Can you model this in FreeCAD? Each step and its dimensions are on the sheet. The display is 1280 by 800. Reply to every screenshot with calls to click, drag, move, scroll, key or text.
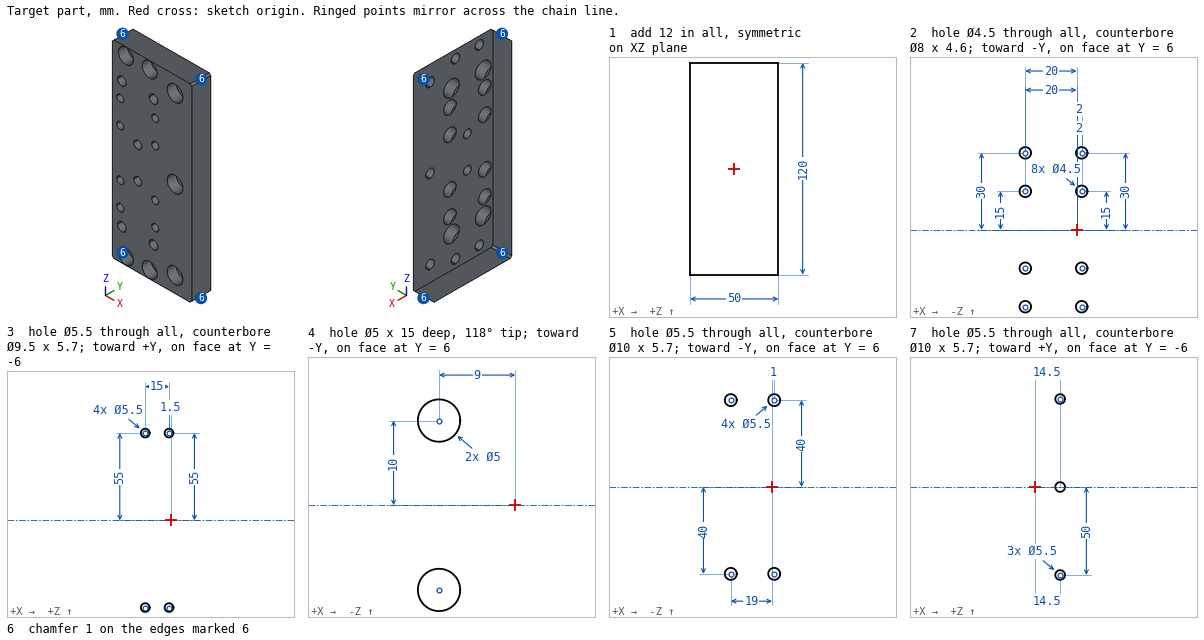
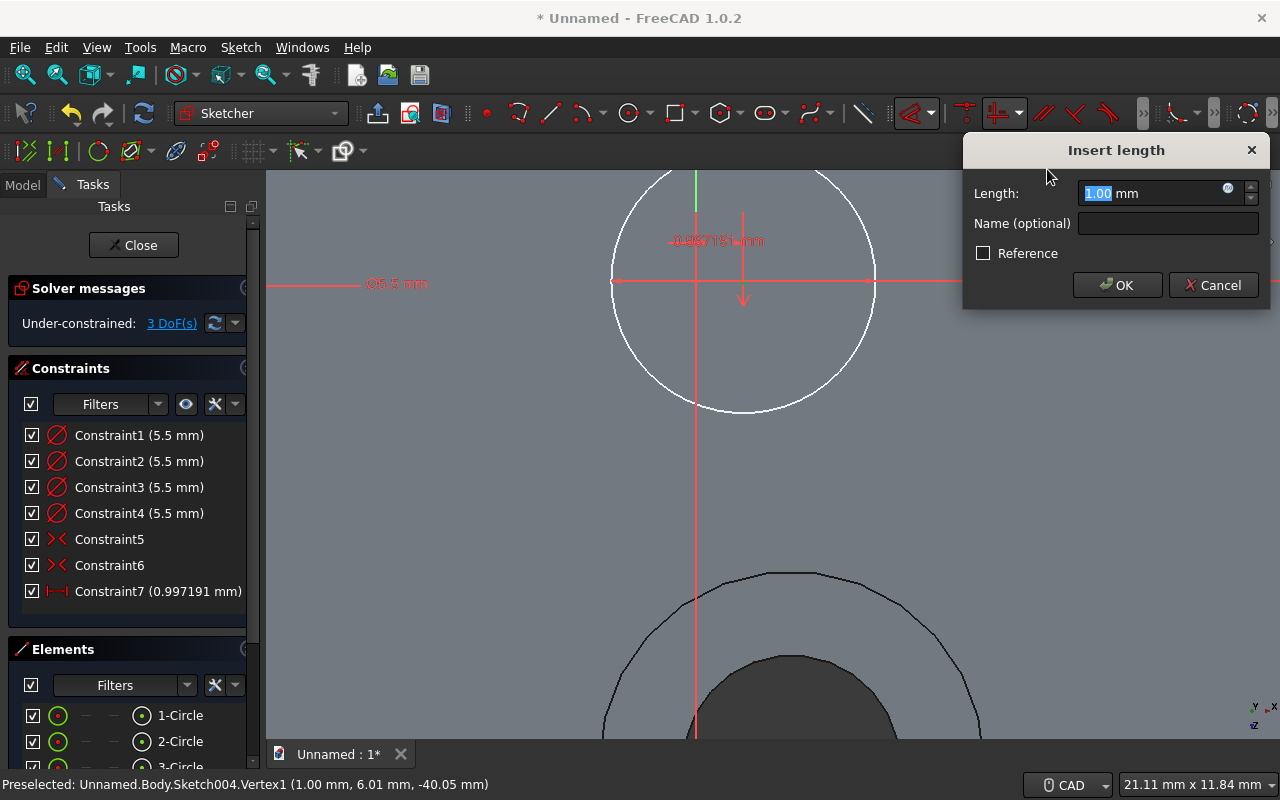
text(1)
key(Return)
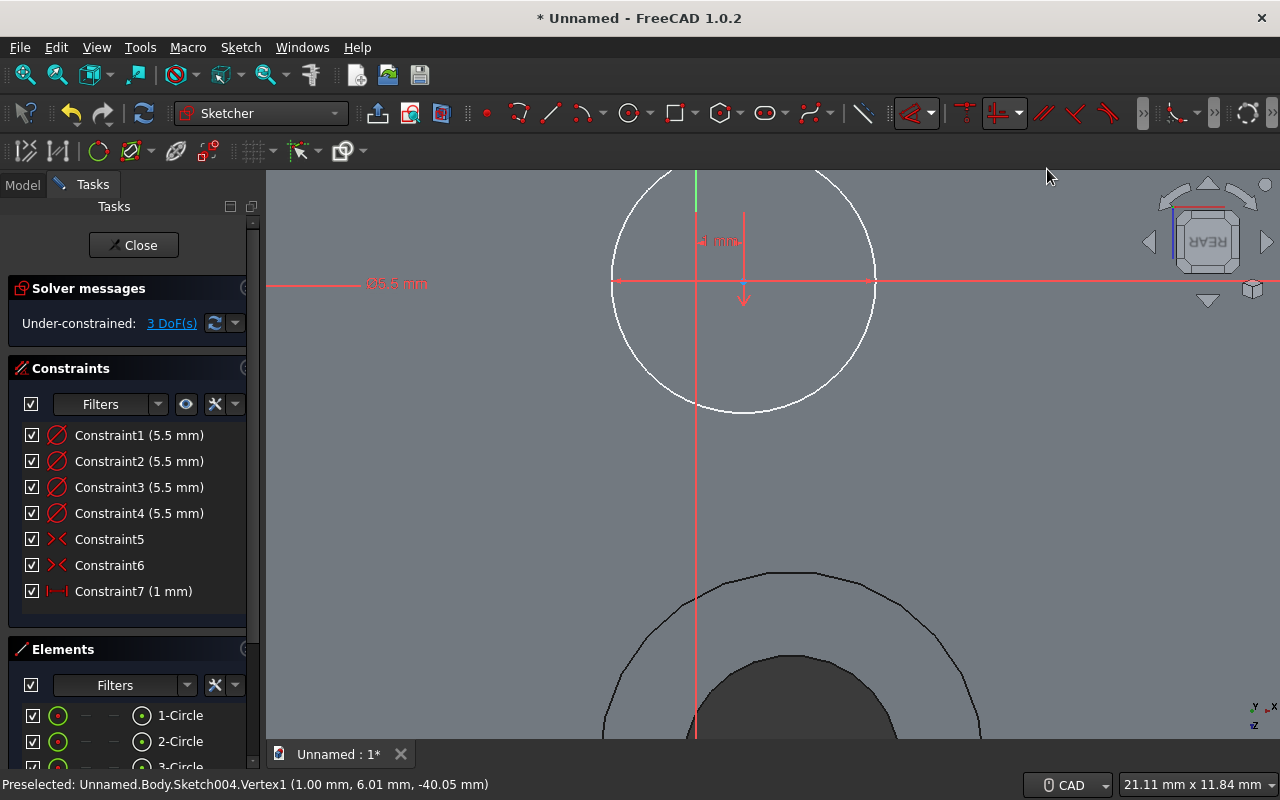
scroll(749, 280, down, 12)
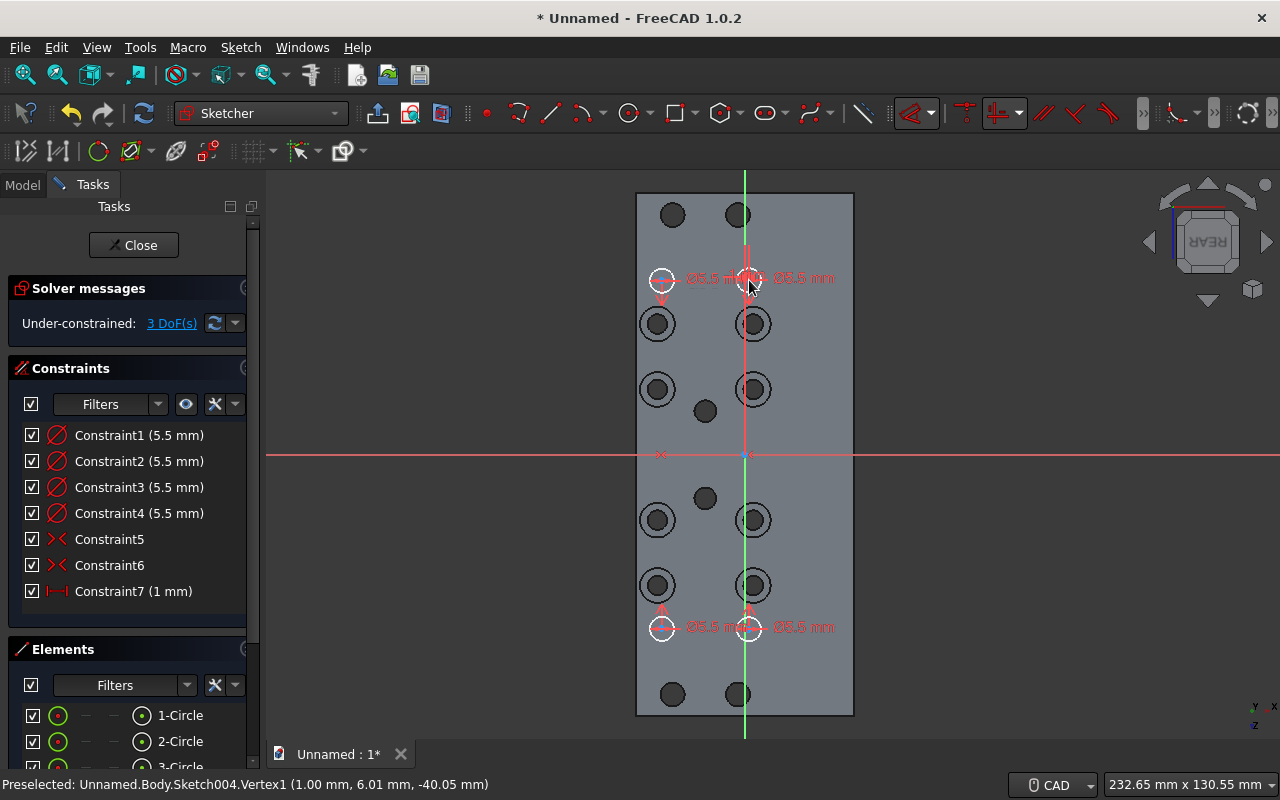
click(749, 280)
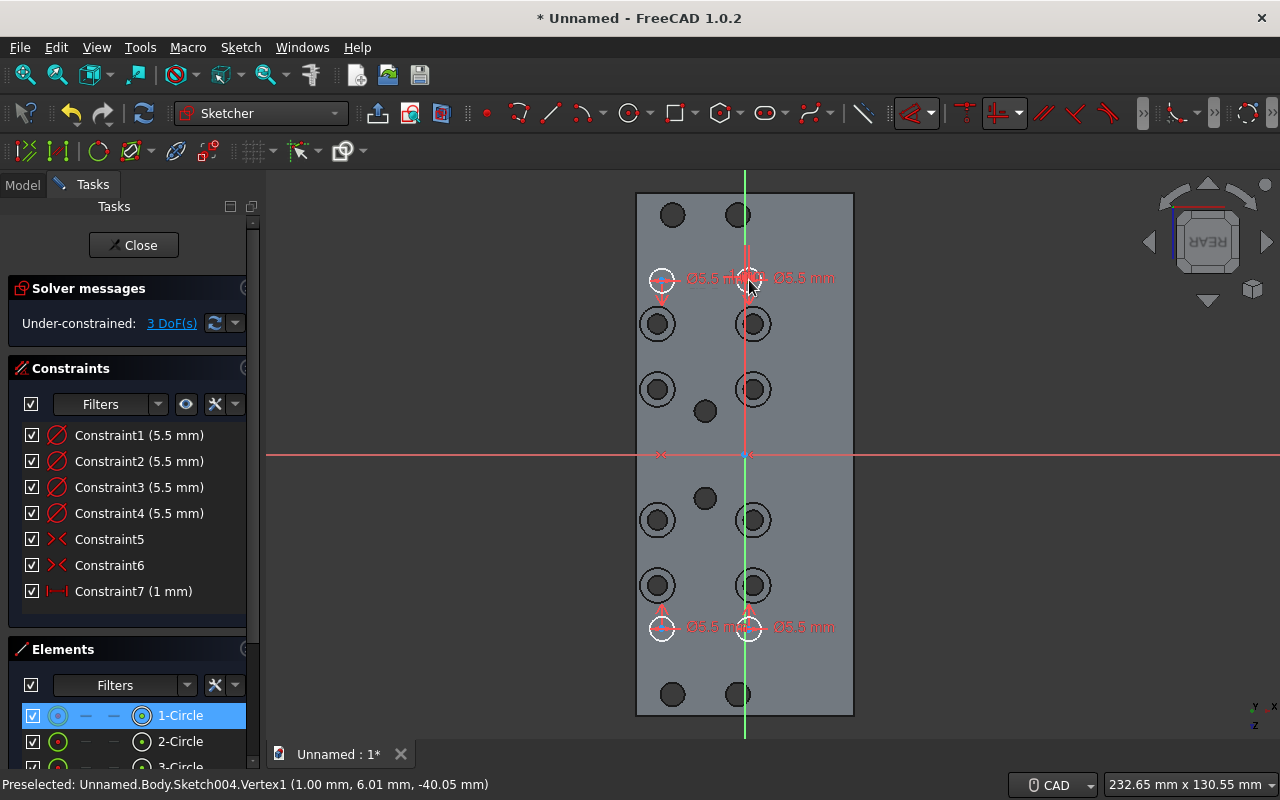
click(934, 114)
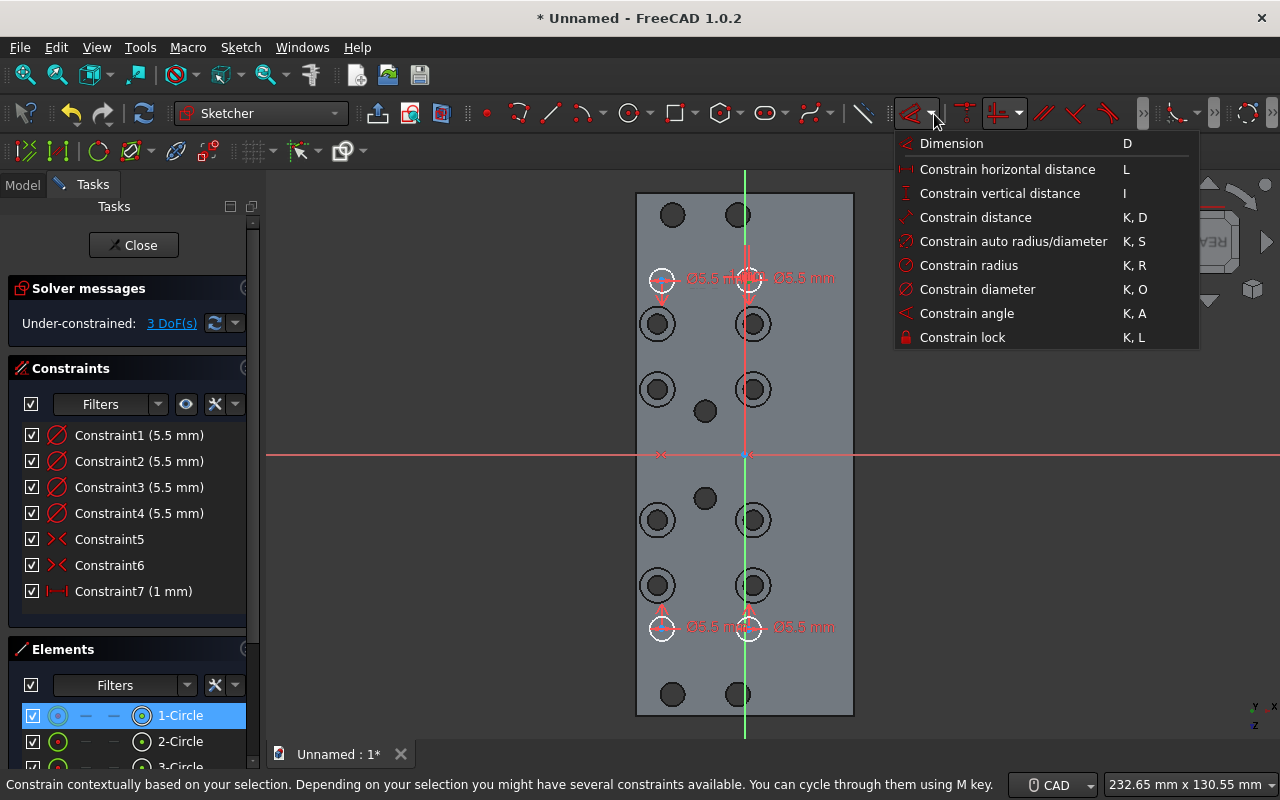
click(1047, 193)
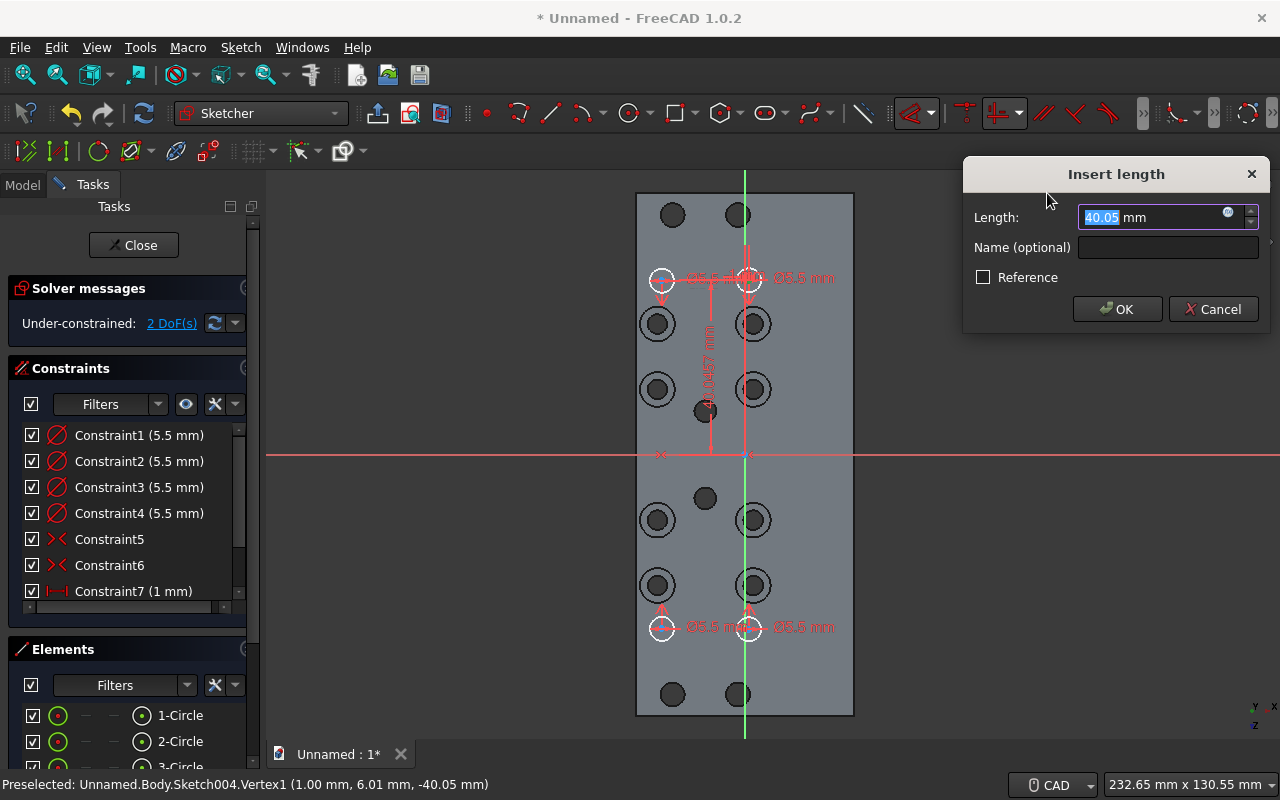
text(40)
key(Return)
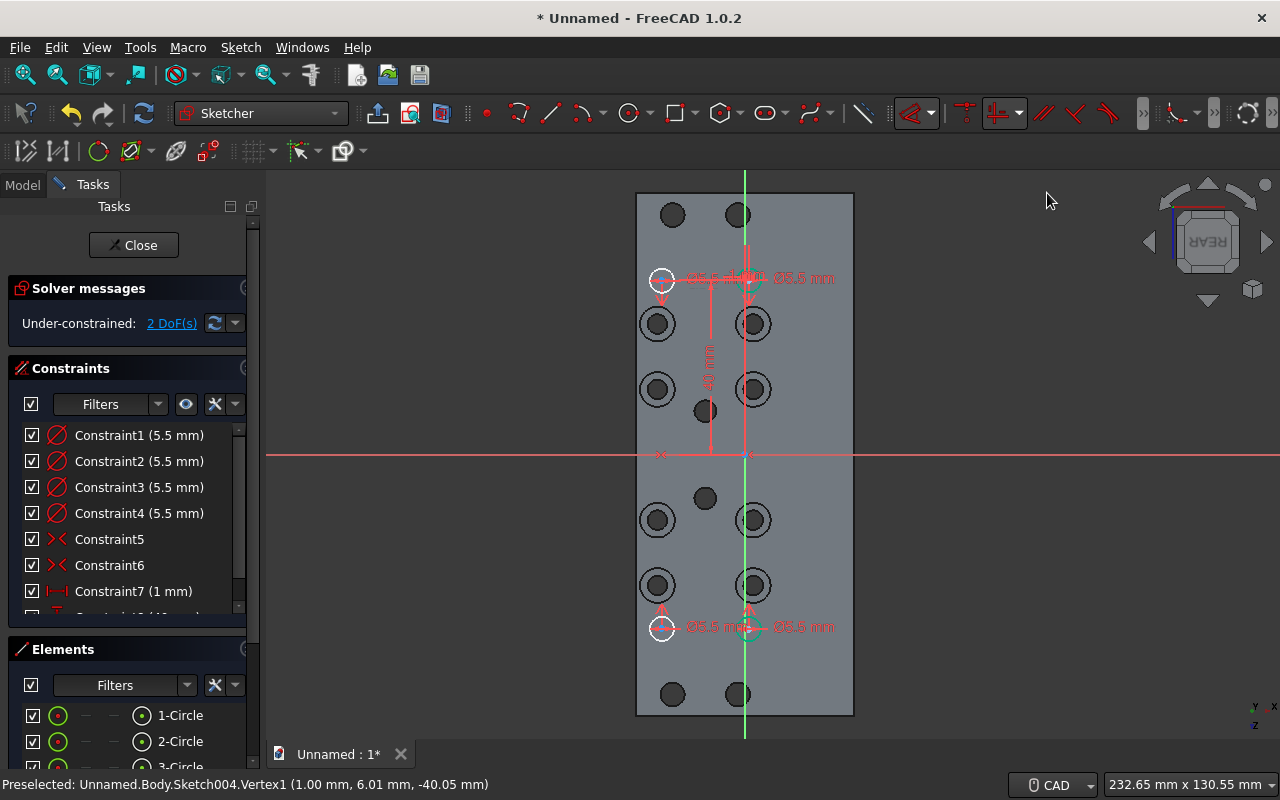
click(662, 629)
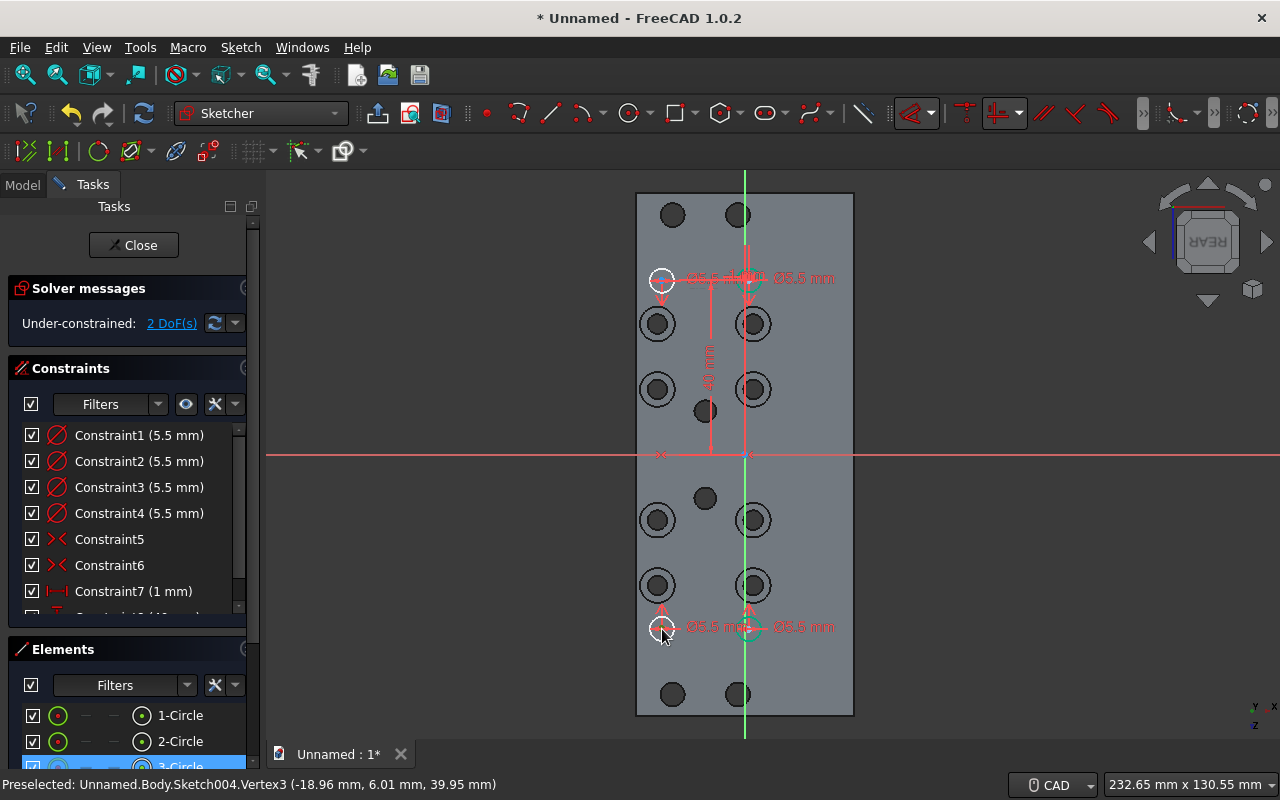
key(l)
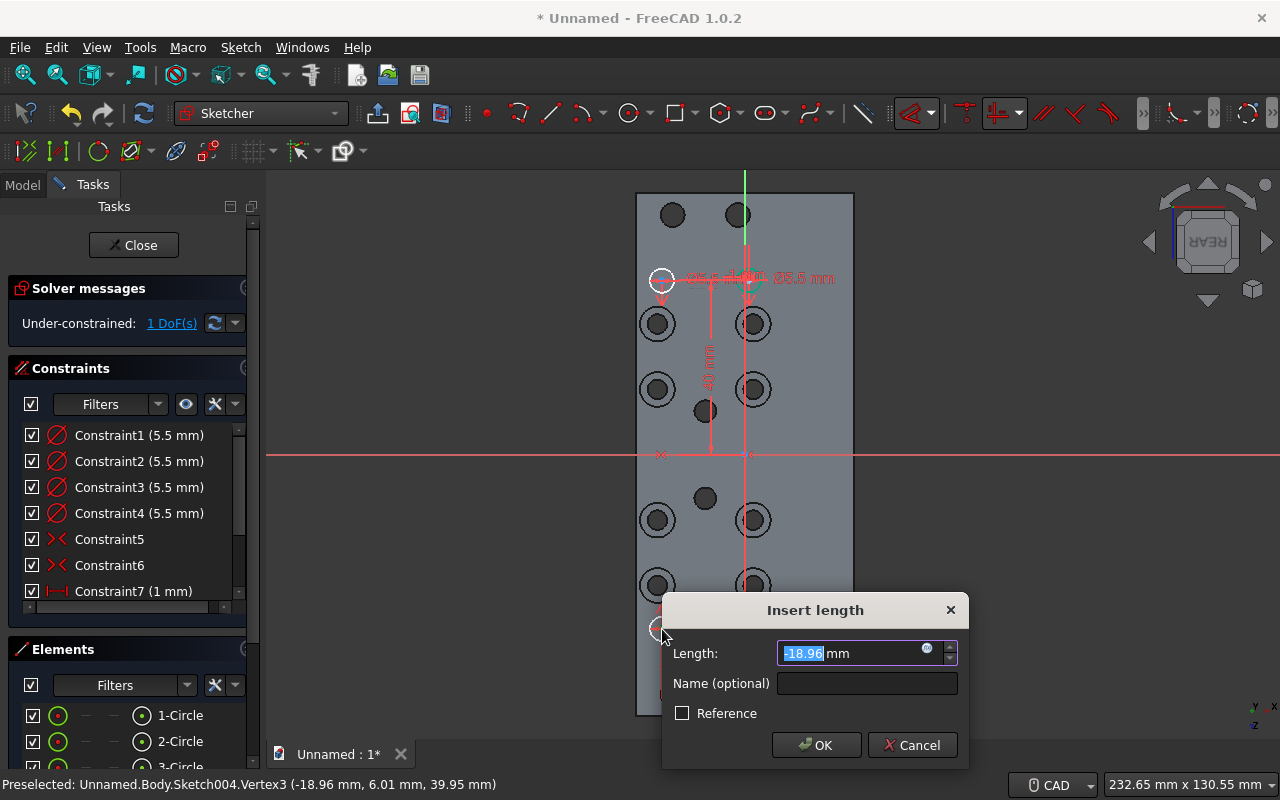
text(-19)
key(Return)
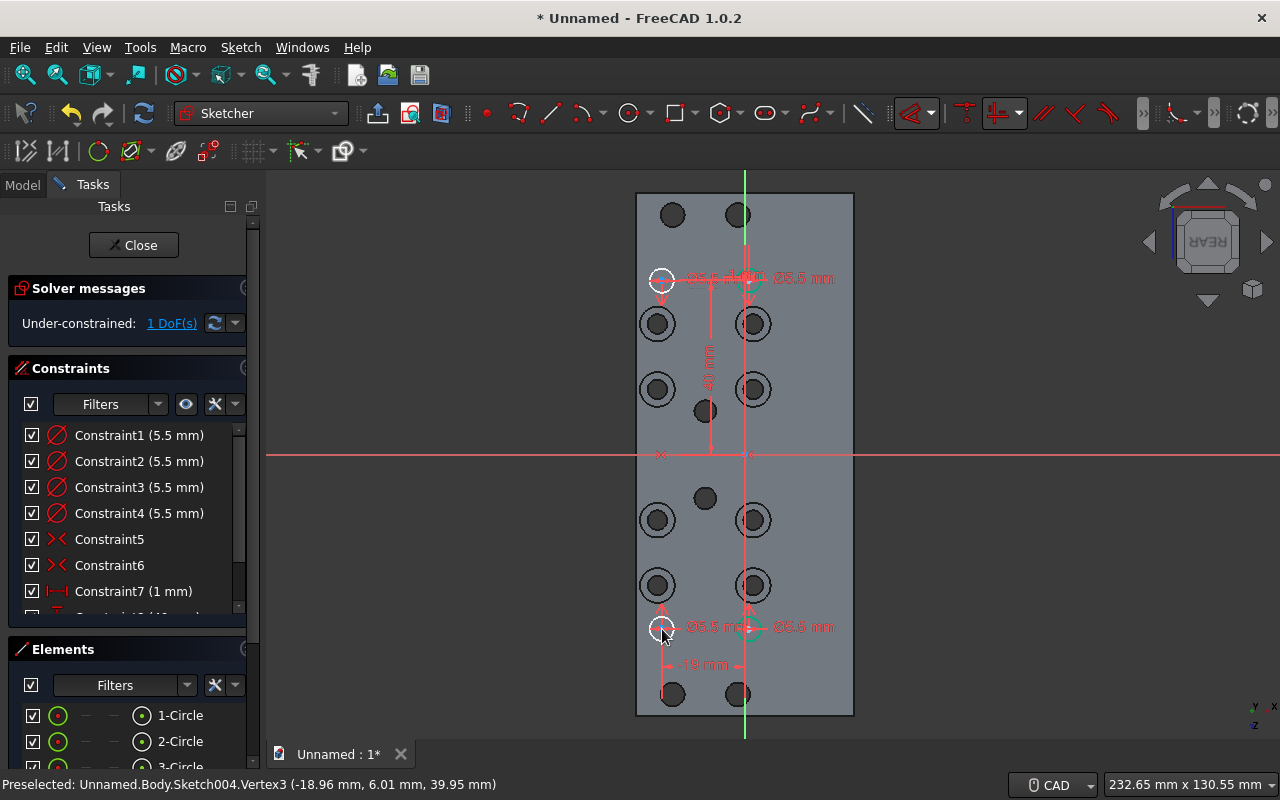
click(662, 629)